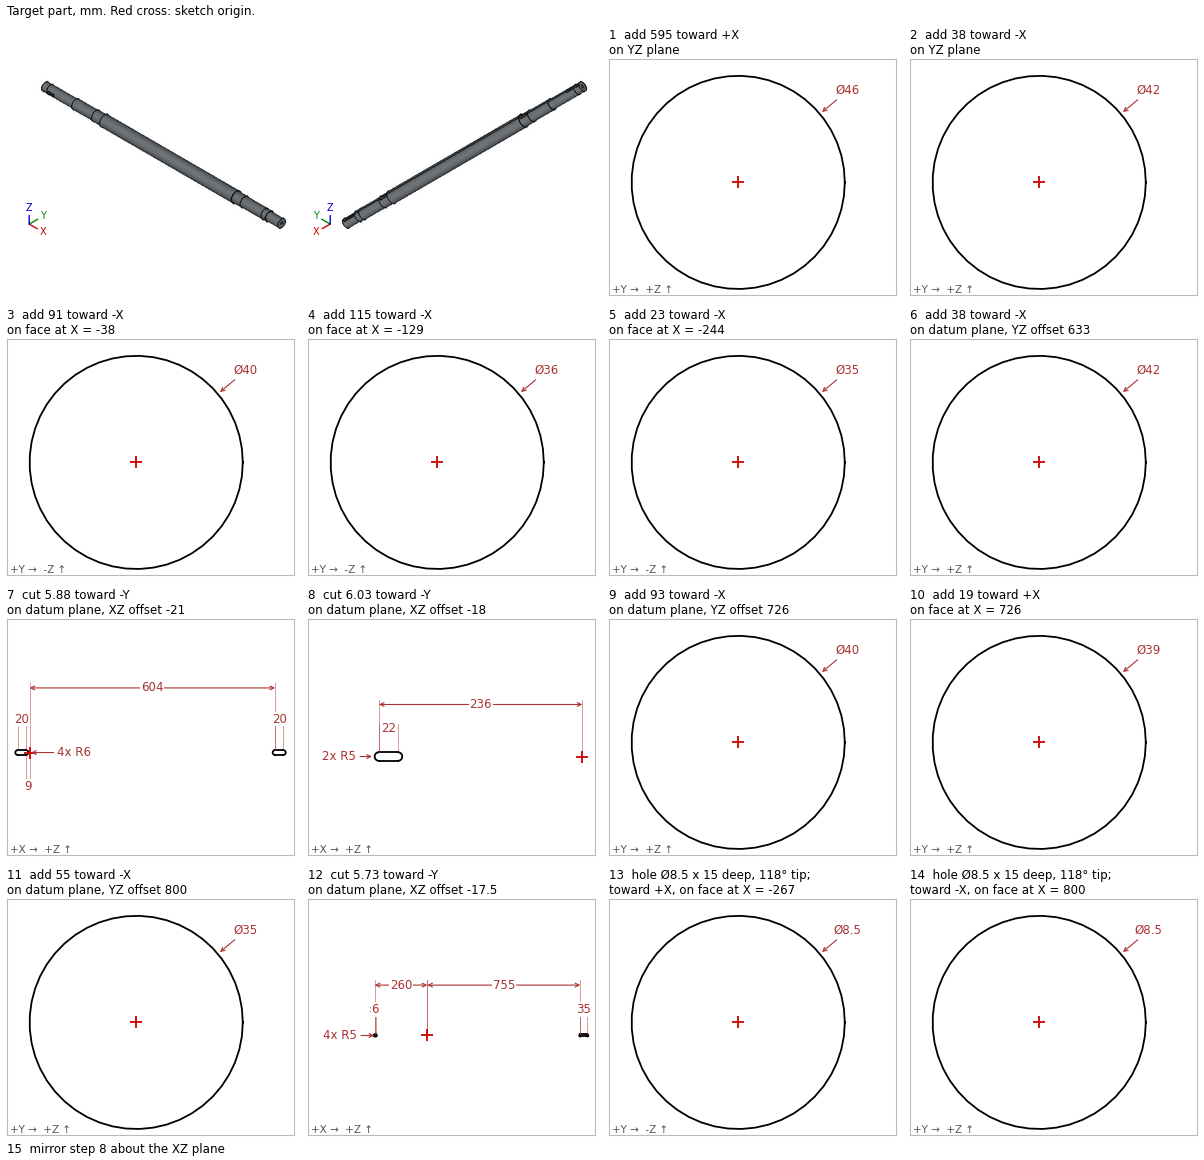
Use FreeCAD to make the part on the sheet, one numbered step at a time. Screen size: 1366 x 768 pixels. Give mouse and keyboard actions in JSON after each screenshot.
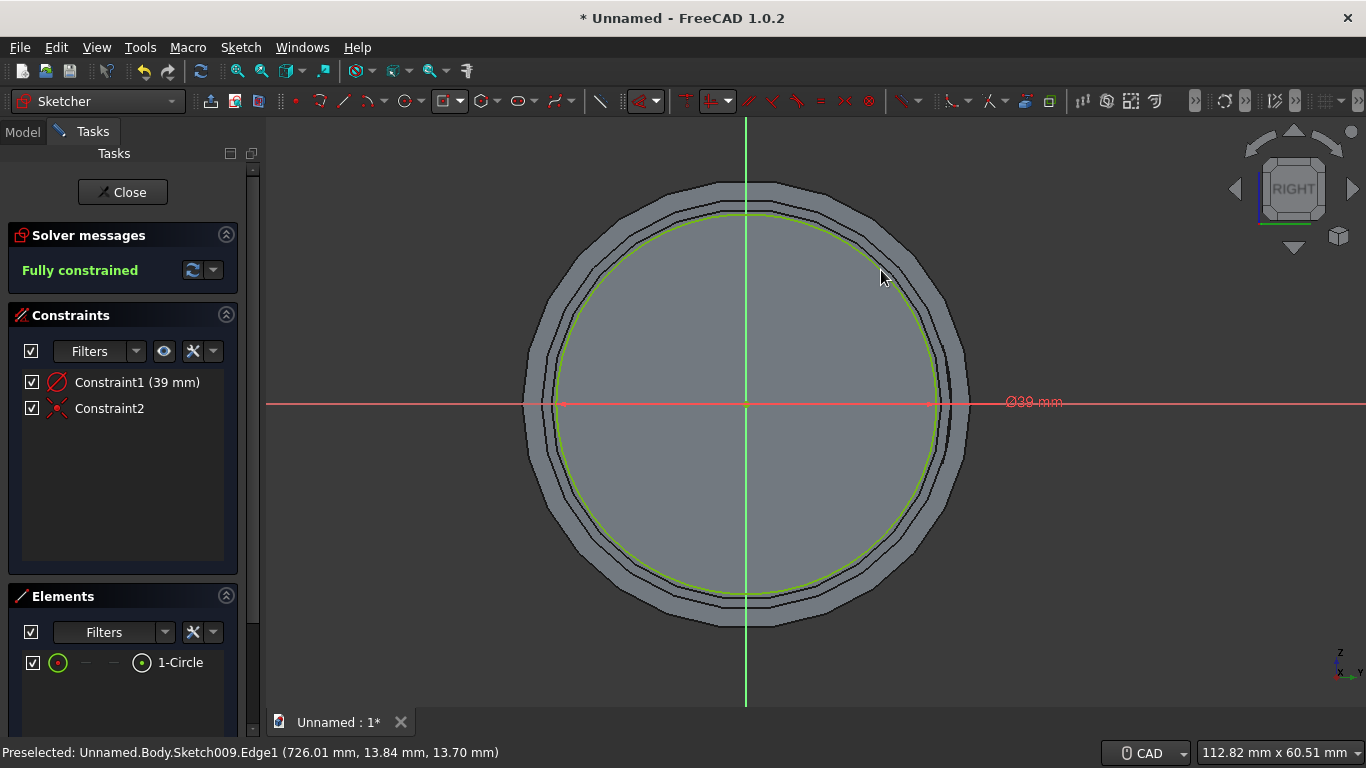
{"action": "left_click", "coordinate": [123, 192]}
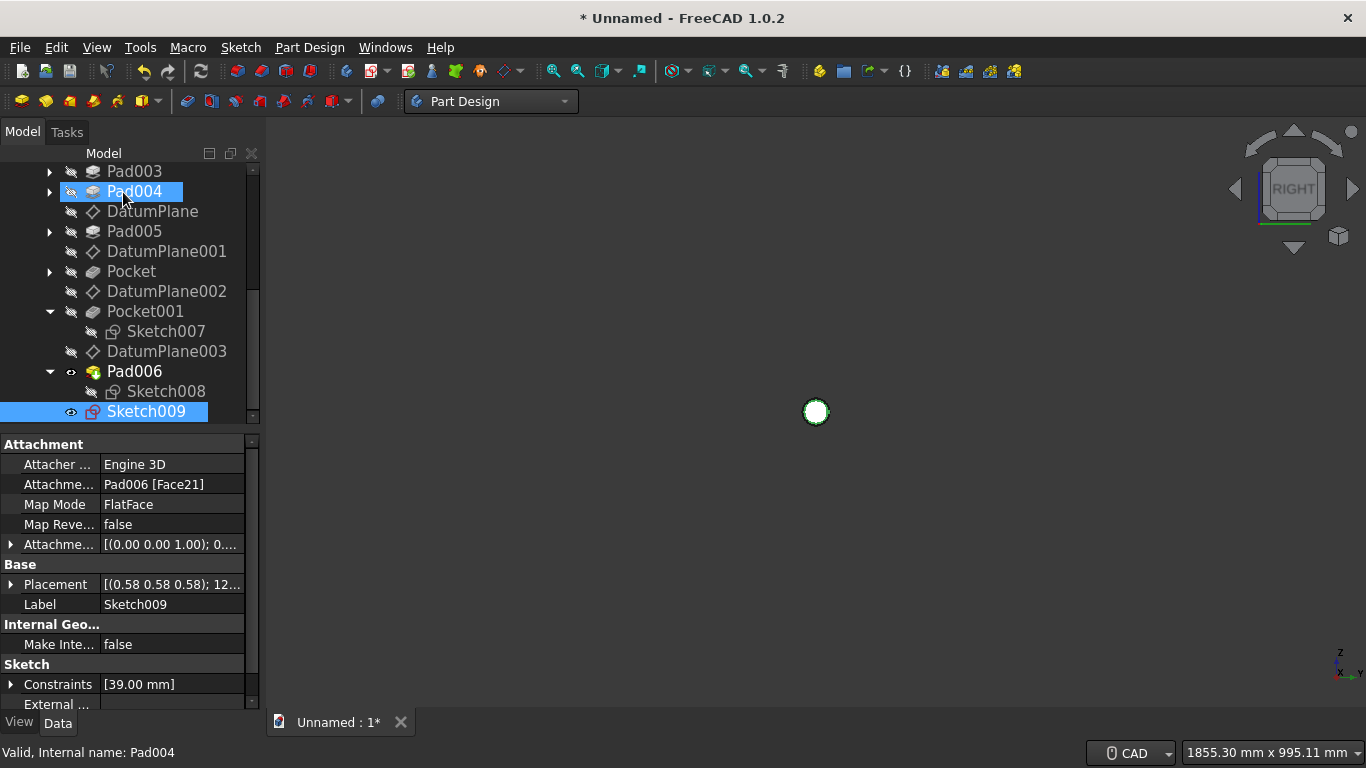
{"action": "left_click", "coordinate": [22, 102]}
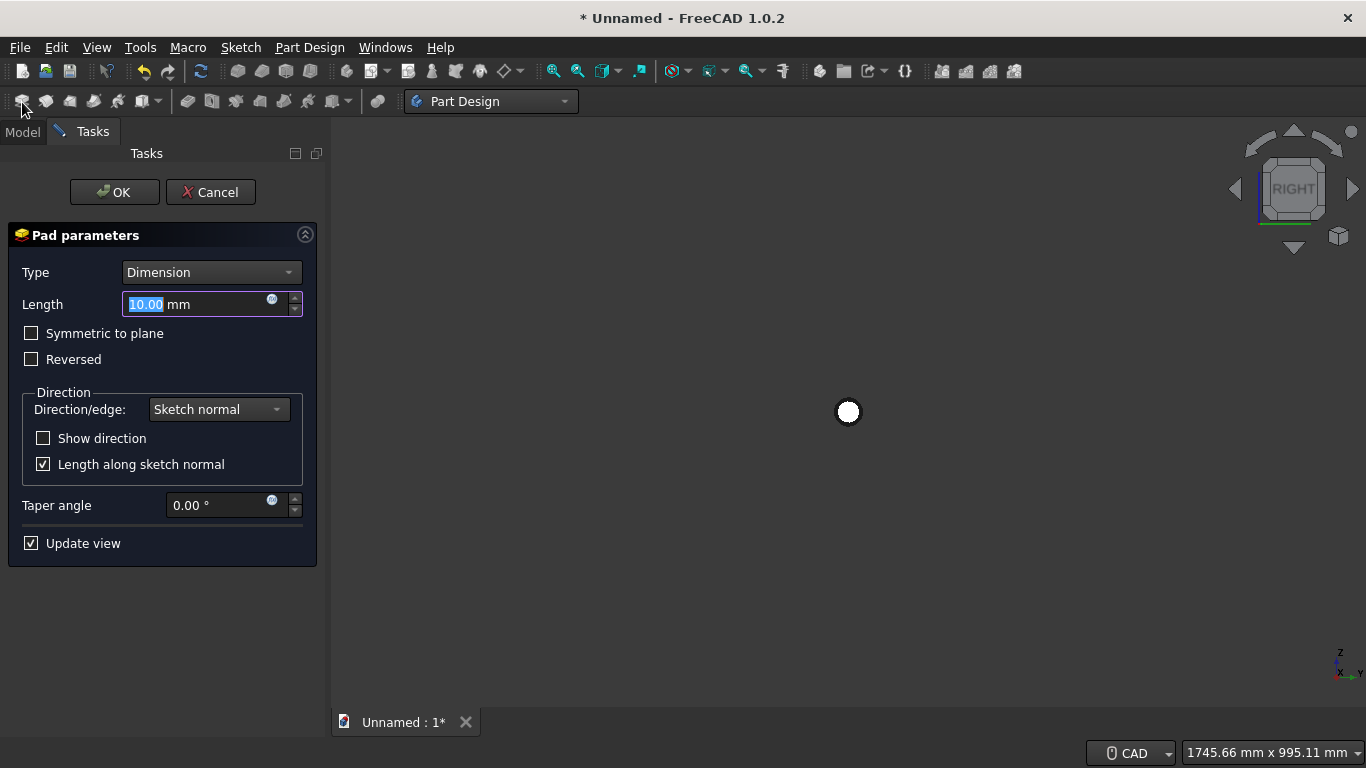
{"action": "type", "text": "19"}
{"action": "key", "text": "Tab"}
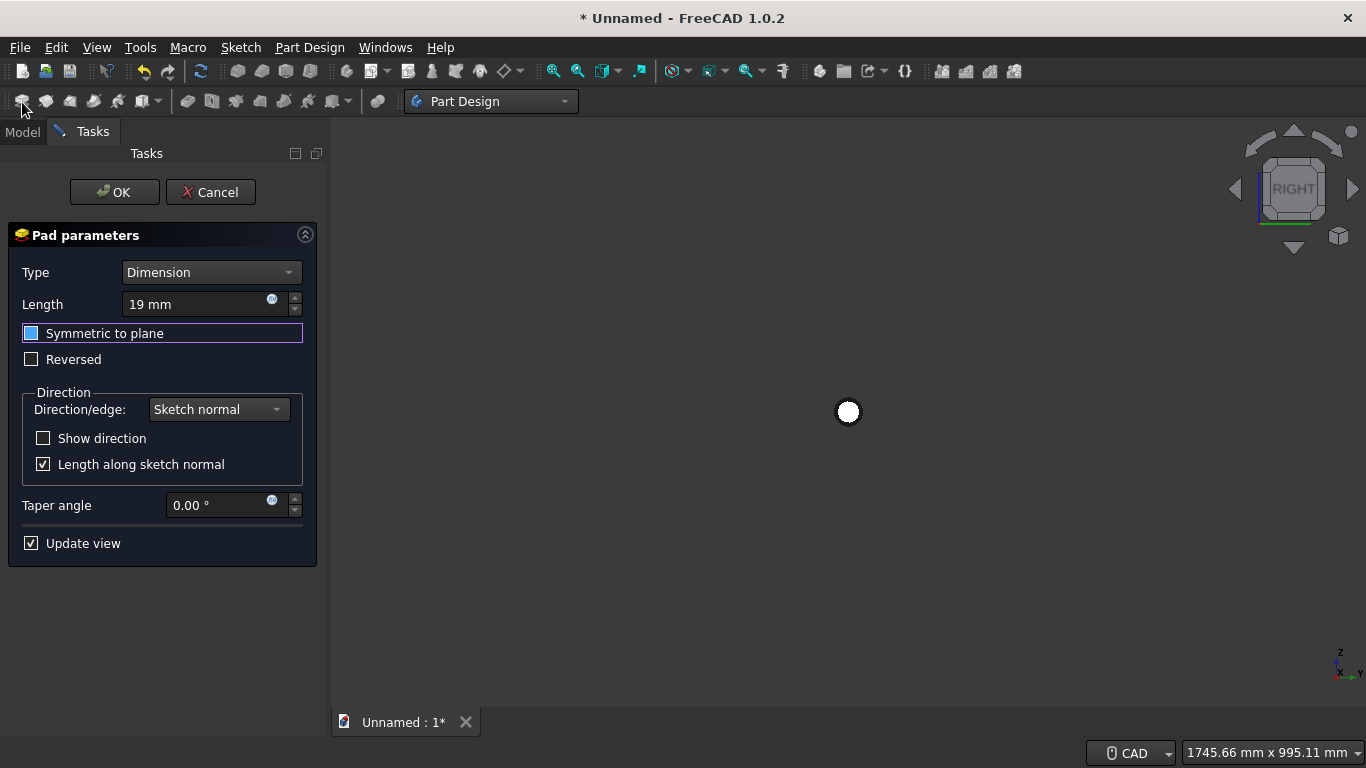
{"action": "left_click", "coordinate": [115, 192]}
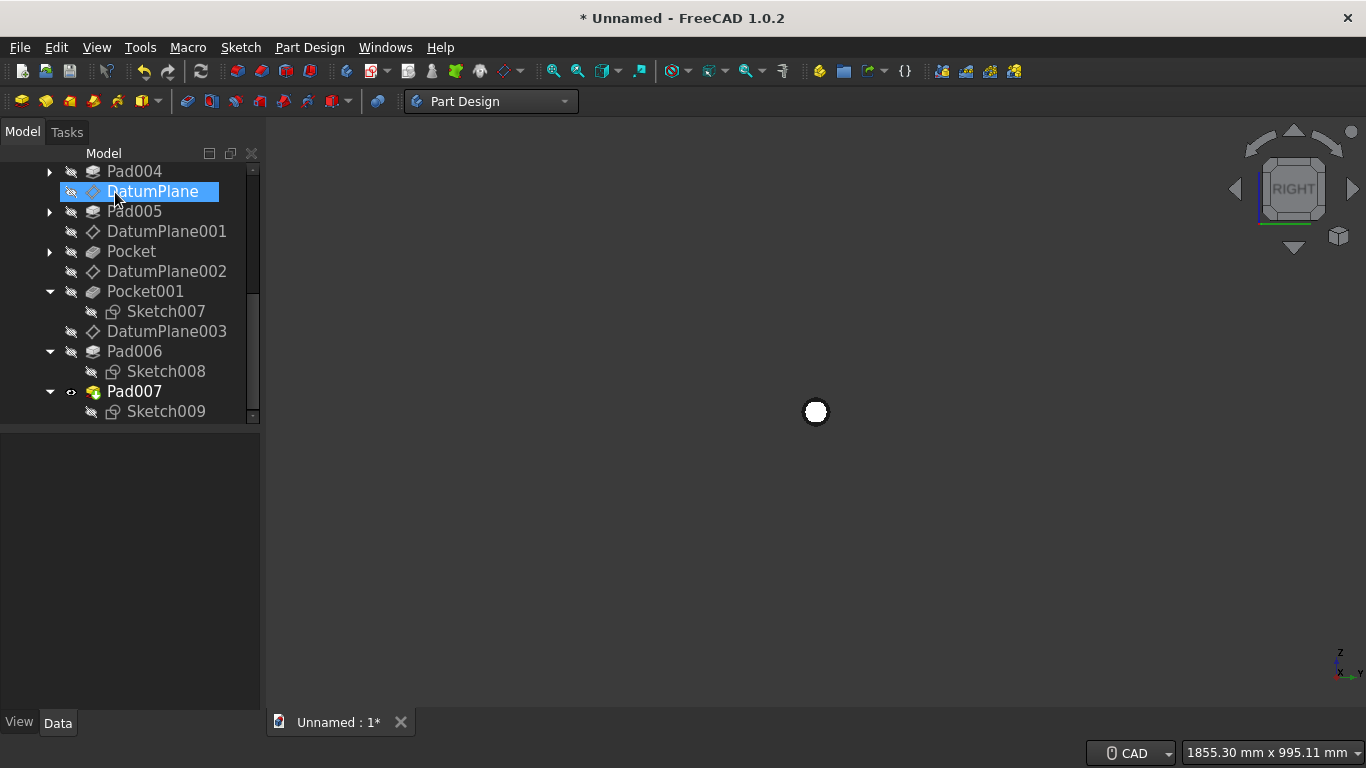
{"action": "key", "text": "v f"}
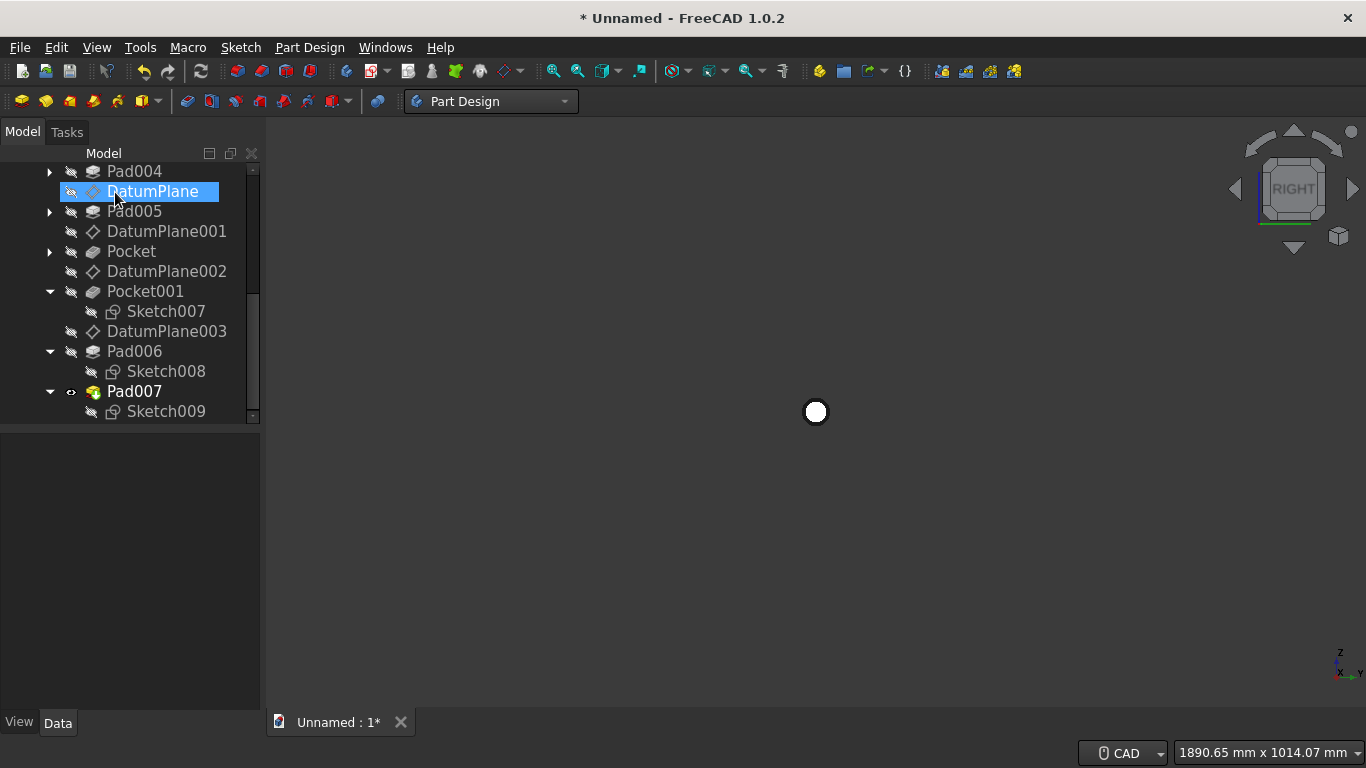
{"action": "scroll", "coordinate": [140, 287], "scroll_direction": "down", "scroll_amount": 3}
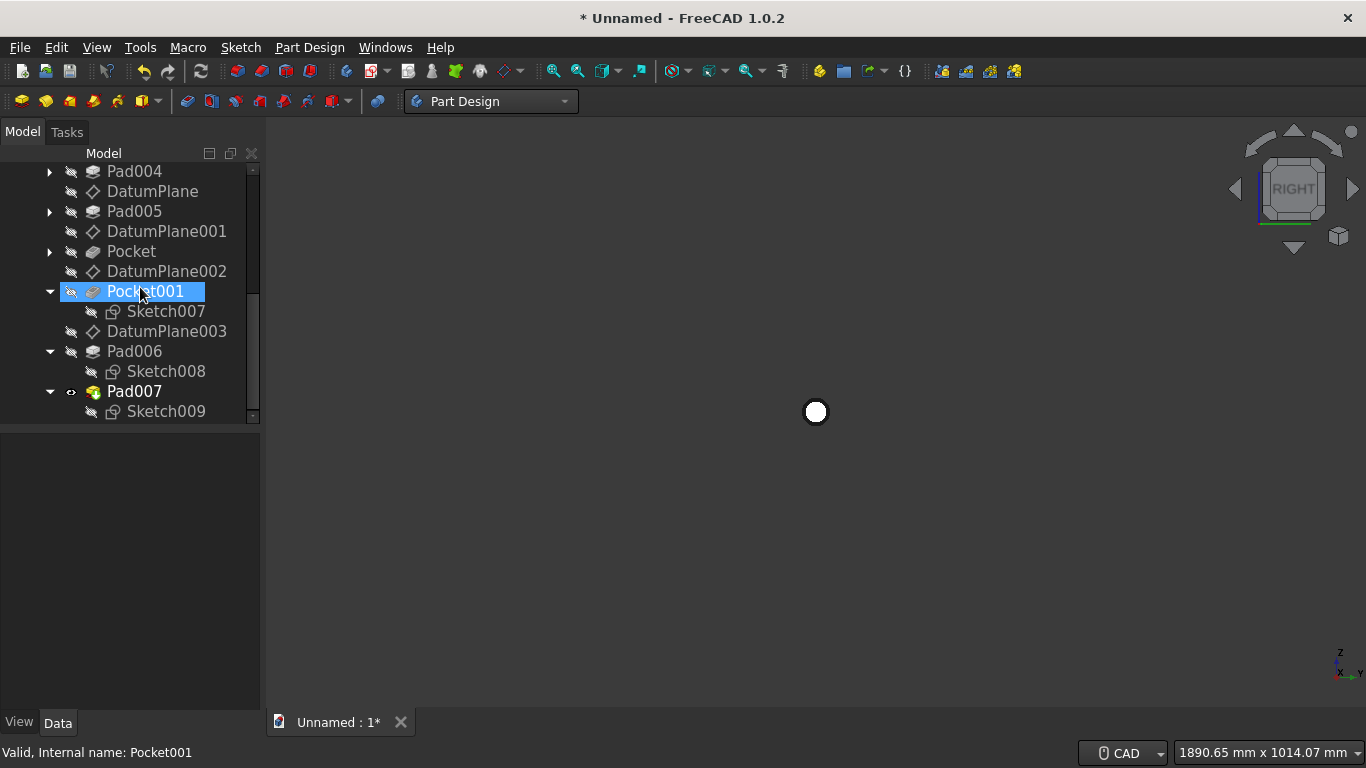
{"action": "scroll", "coordinate": [140, 287], "scroll_direction": "up", "scroll_amount": 15}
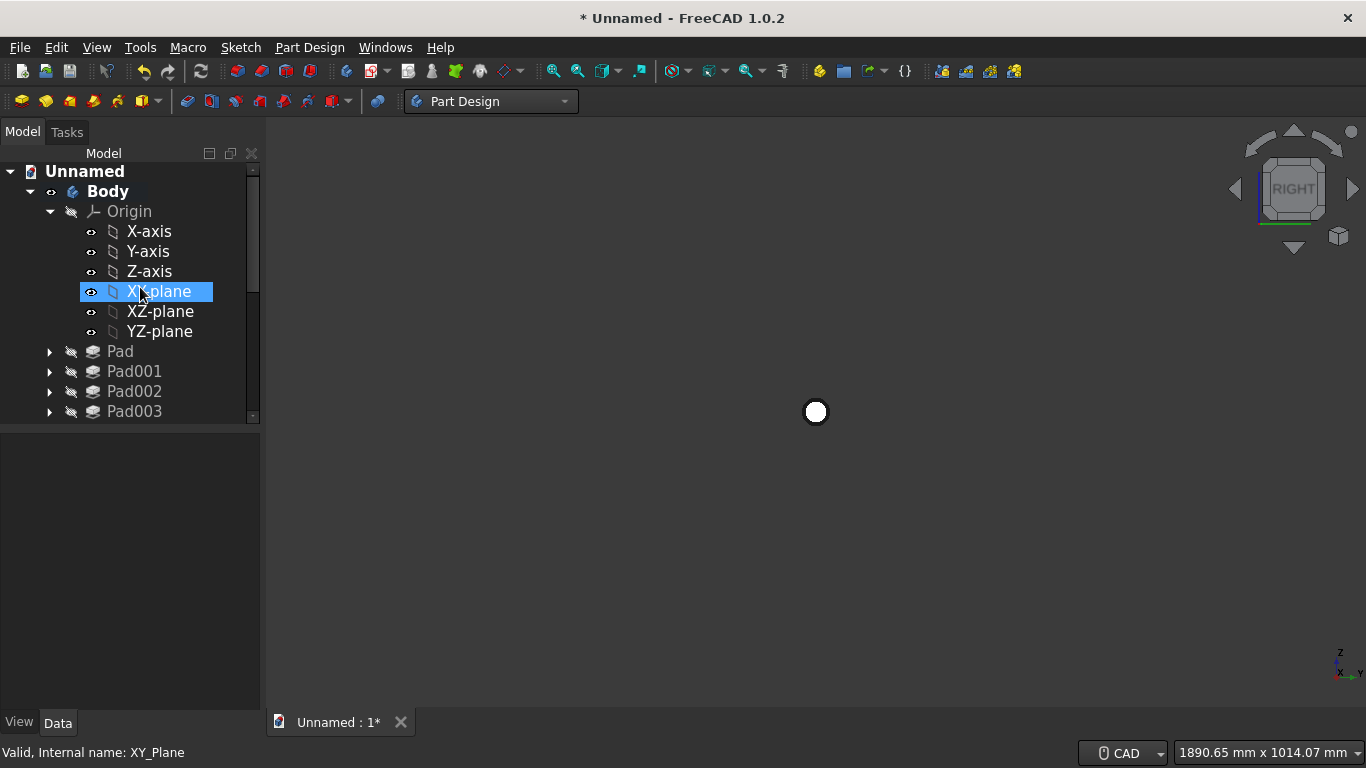
{"action": "left_click", "coordinate": [136, 332]}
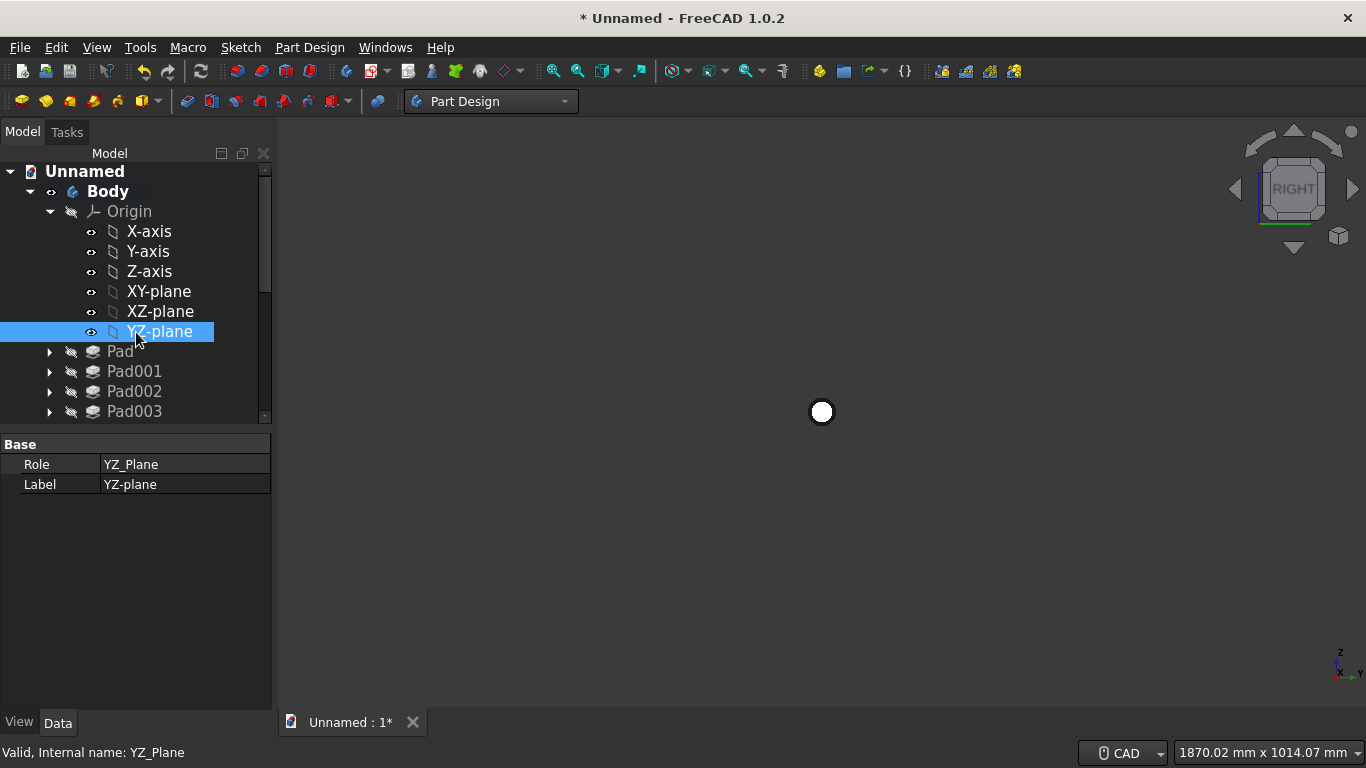
{"action": "left_click", "coordinate": [504, 72]}